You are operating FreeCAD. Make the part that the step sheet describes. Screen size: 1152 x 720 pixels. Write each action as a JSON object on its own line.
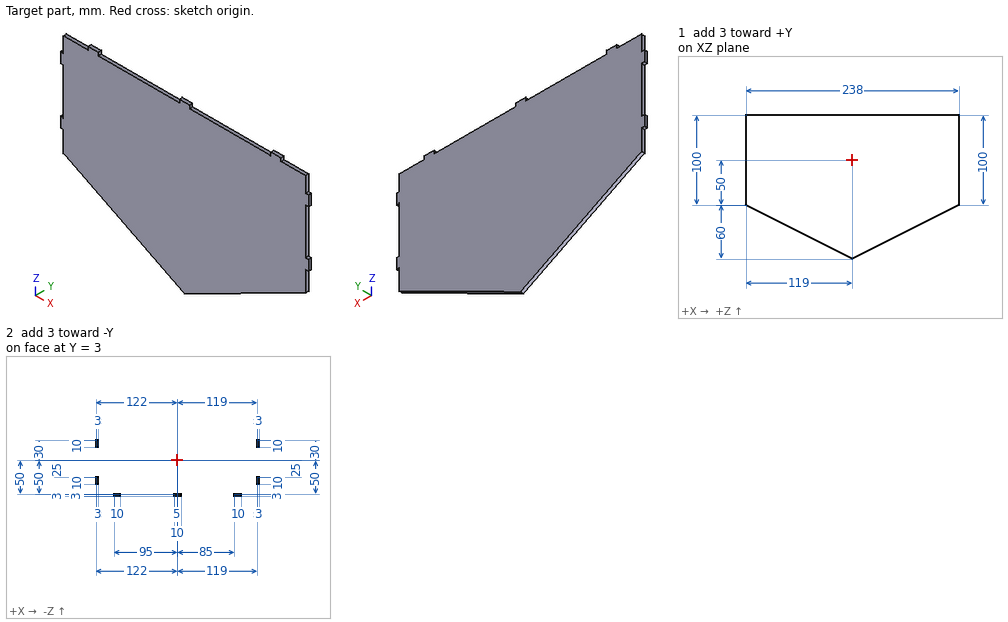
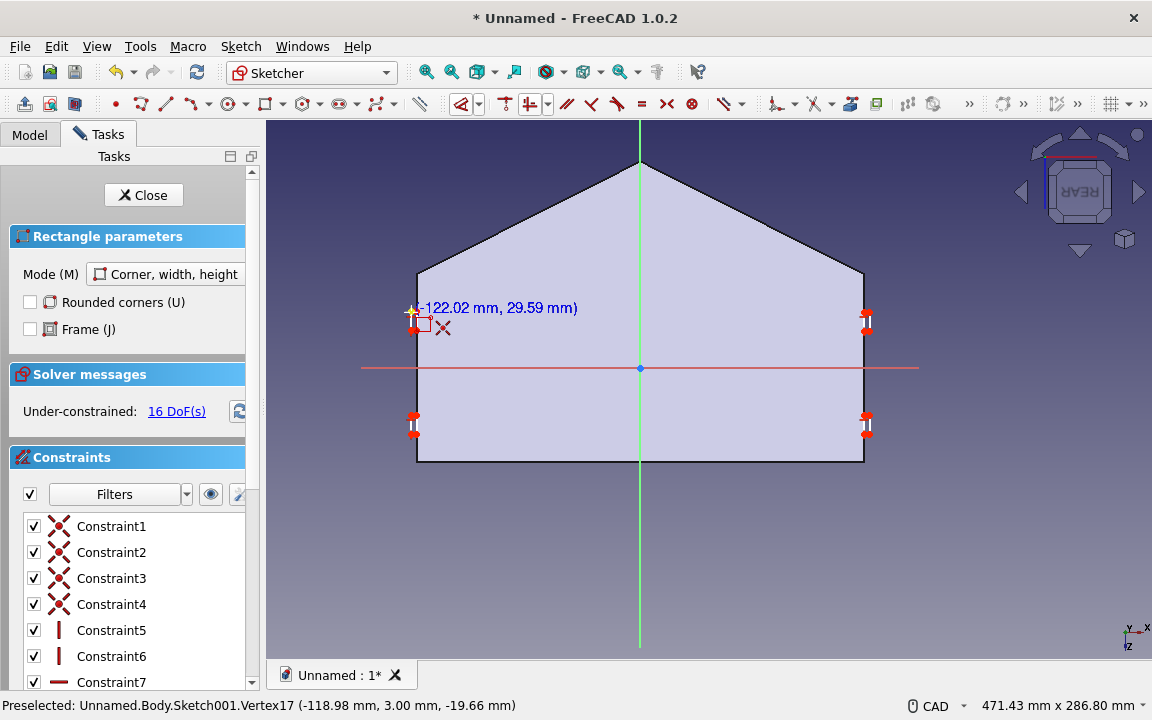
{"action": "scroll", "coordinate": [462, 462], "scroll_direction": "up", "scroll_amount": 6}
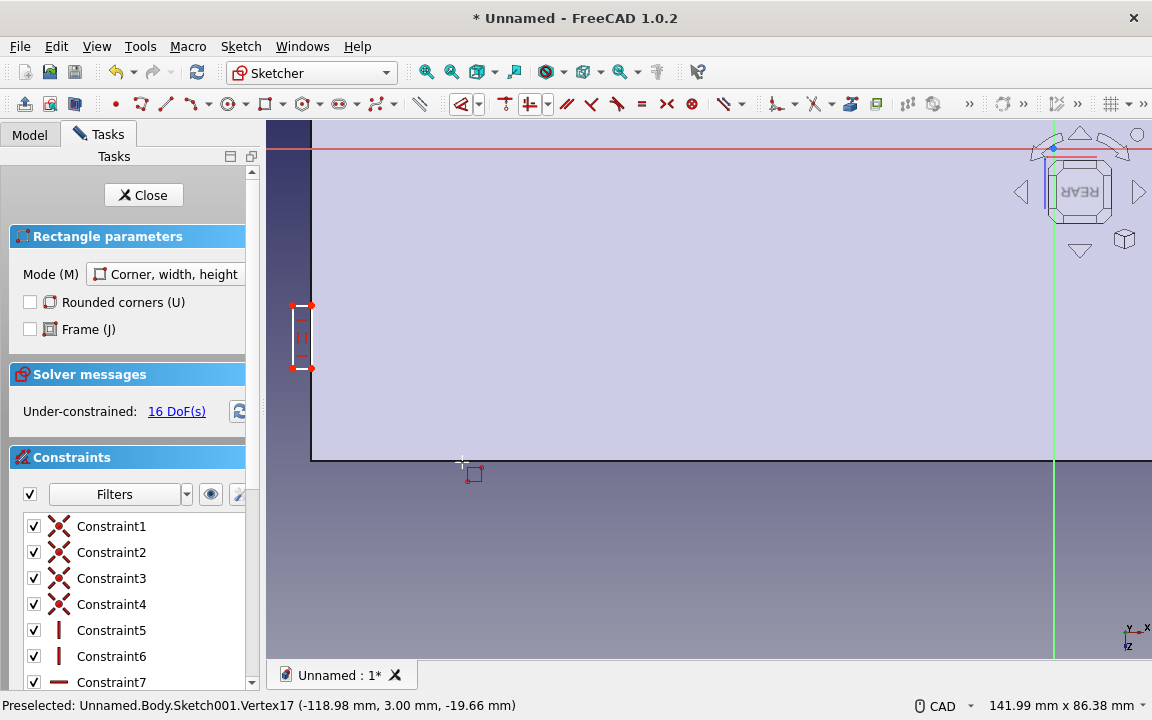
{"action": "left_click", "coordinate": [461, 461]}
{"action": "left_click", "coordinate": [524, 480]}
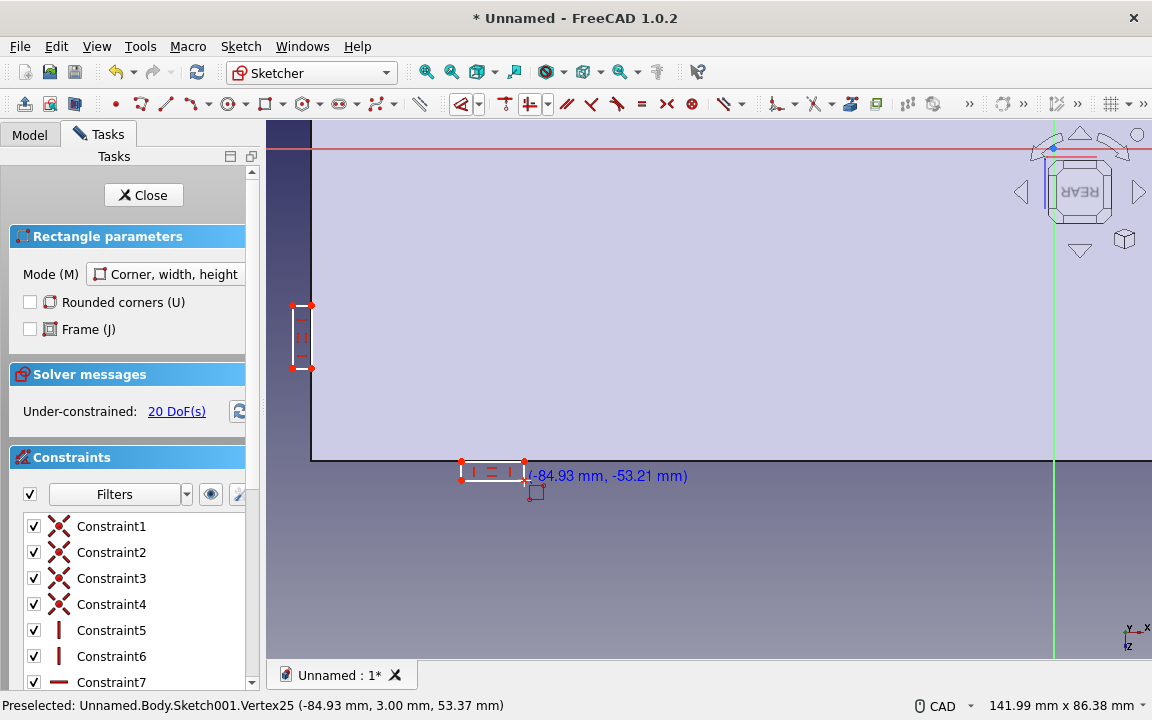
{"action": "scroll", "coordinate": [462, 462], "scroll_direction": "down", "scroll_amount": 6}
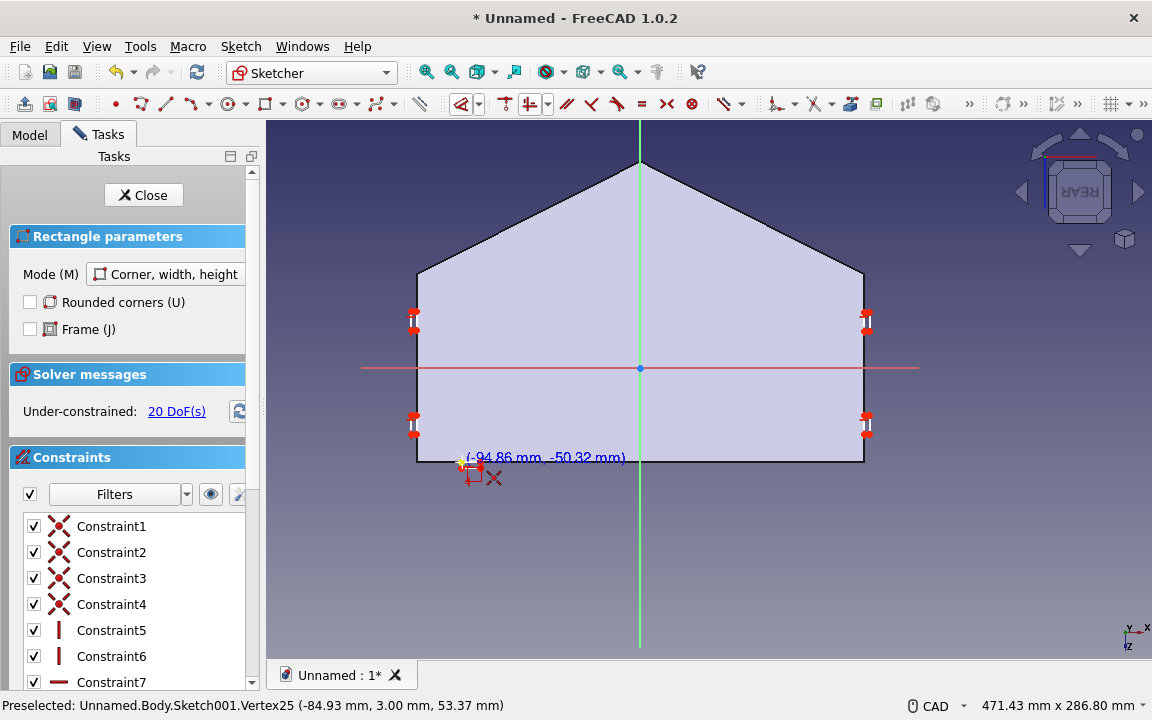
{"action": "scroll", "coordinate": [800, 462], "scroll_direction": "up", "scroll_amount": 6}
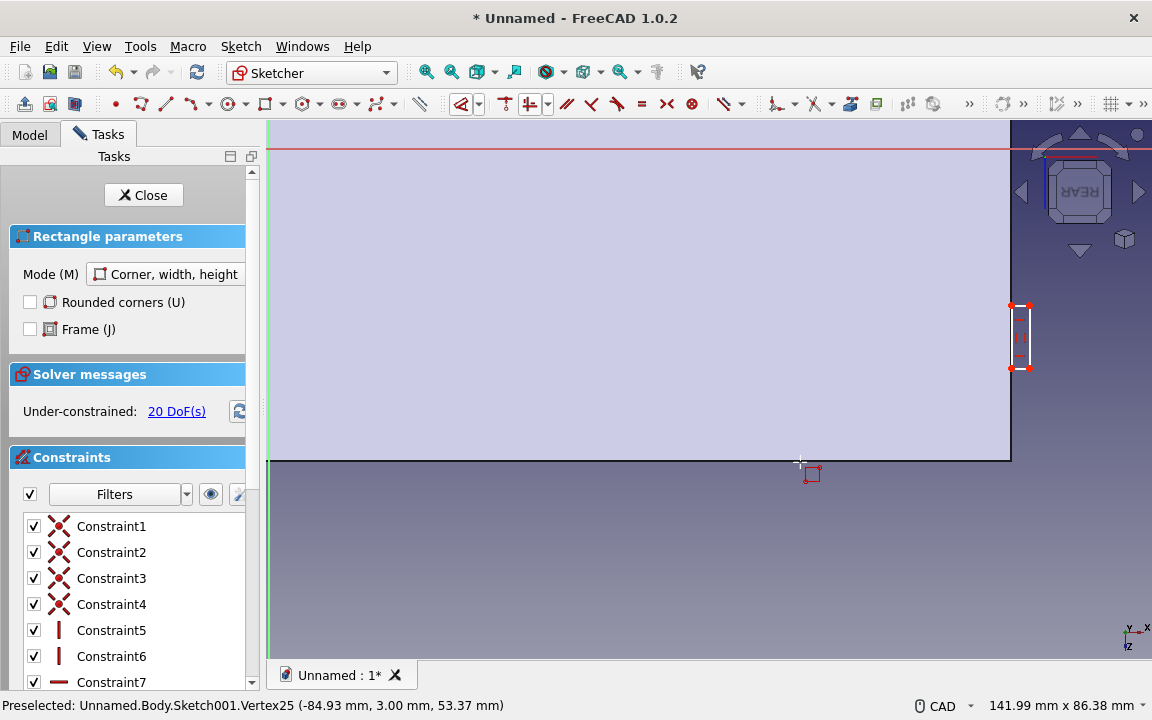
{"action": "left_click", "coordinate": [799, 461]}
{"action": "left_click", "coordinate": [862, 480]}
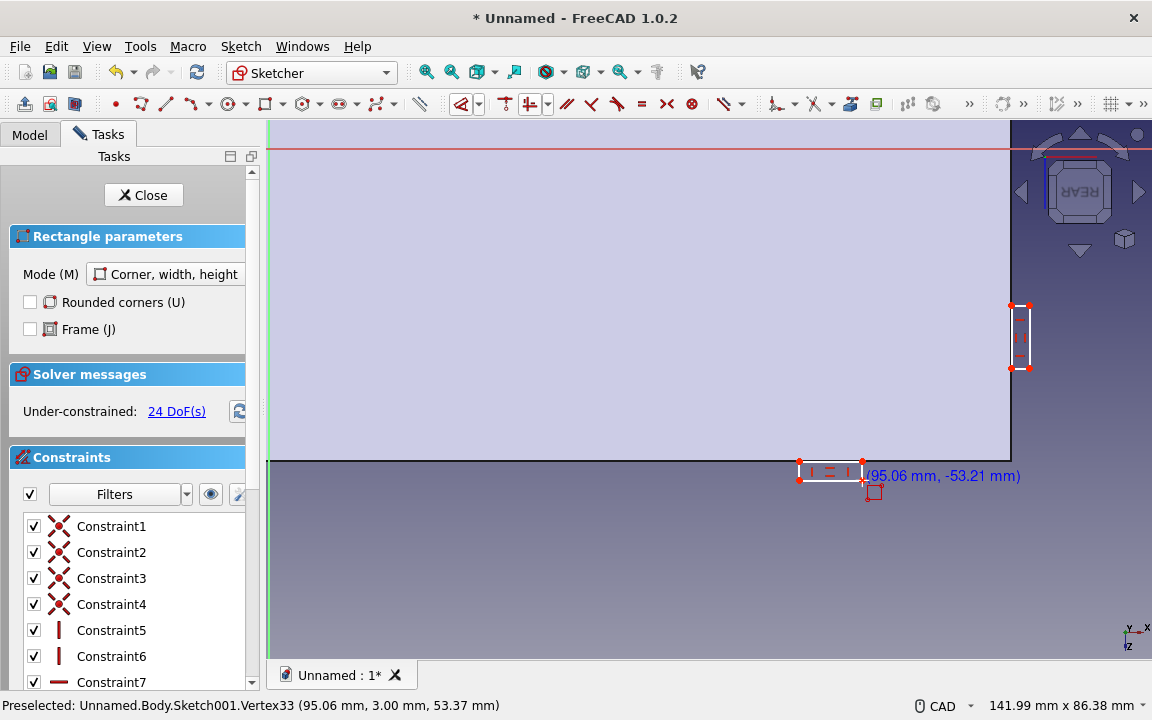
{"action": "scroll", "coordinate": [801, 462], "scroll_direction": "down", "scroll_amount": 6}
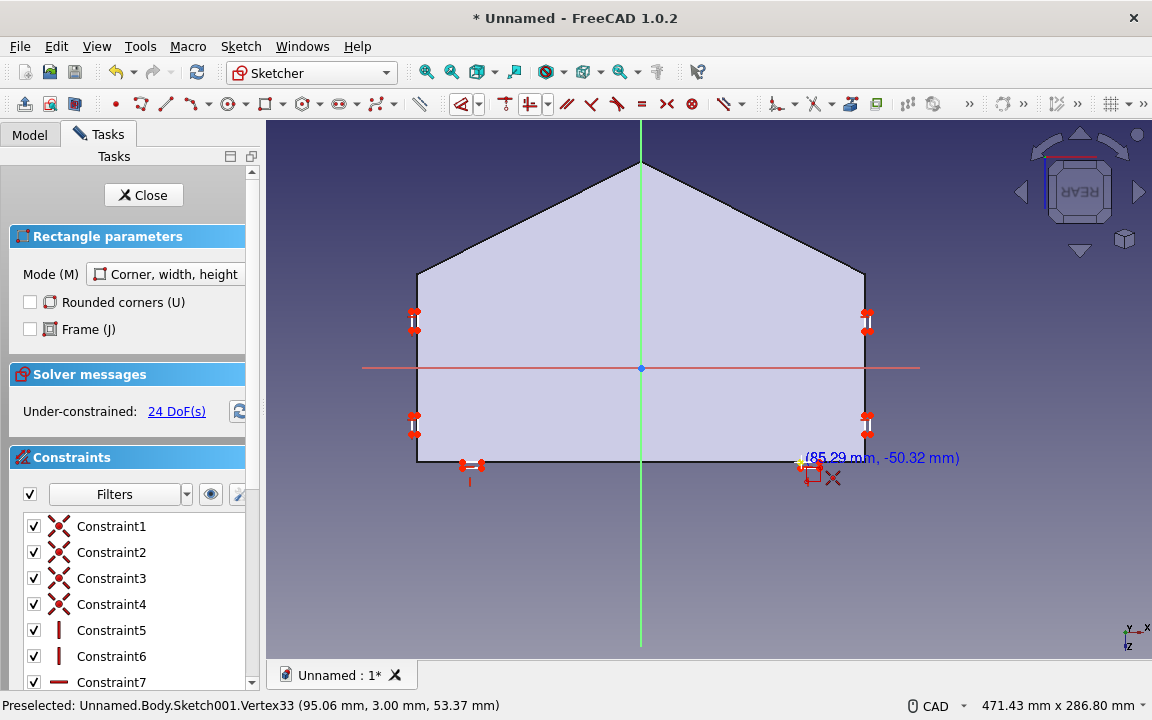
{"action": "scroll", "coordinate": [632, 462], "scroll_direction": "up", "scroll_amount": 6}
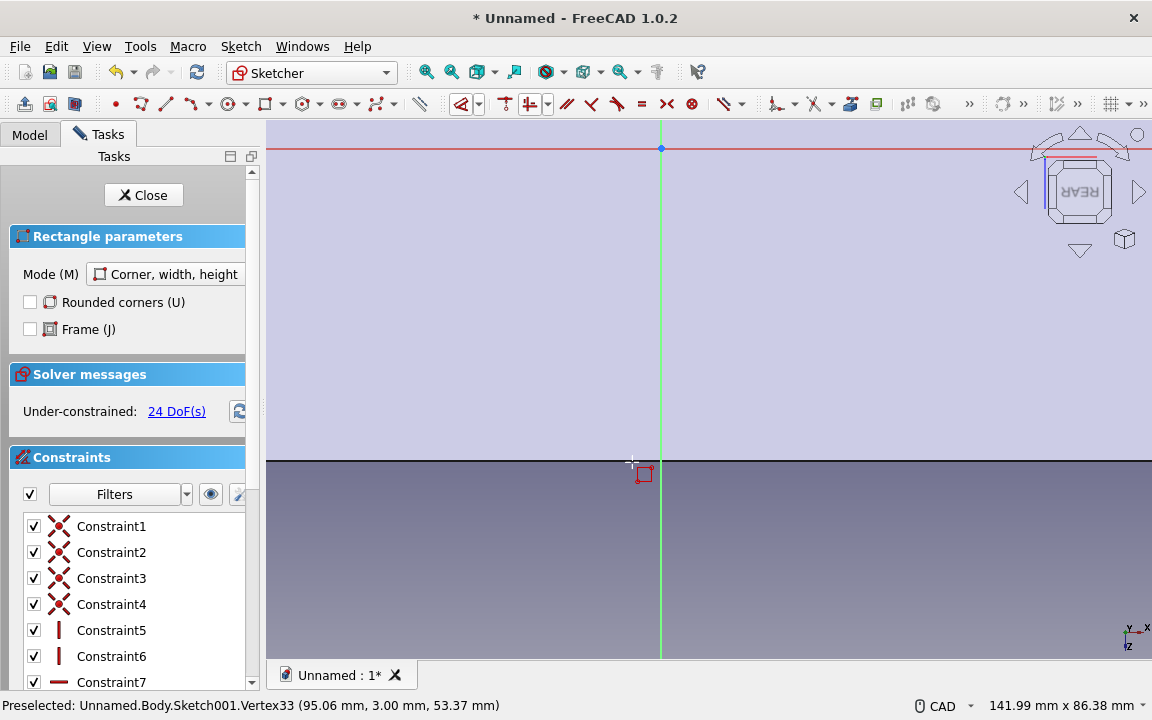
{"action": "left_click", "coordinate": [630, 461]}
{"action": "left_click", "coordinate": [693, 480]}
{"action": "key", "text": "Escape"}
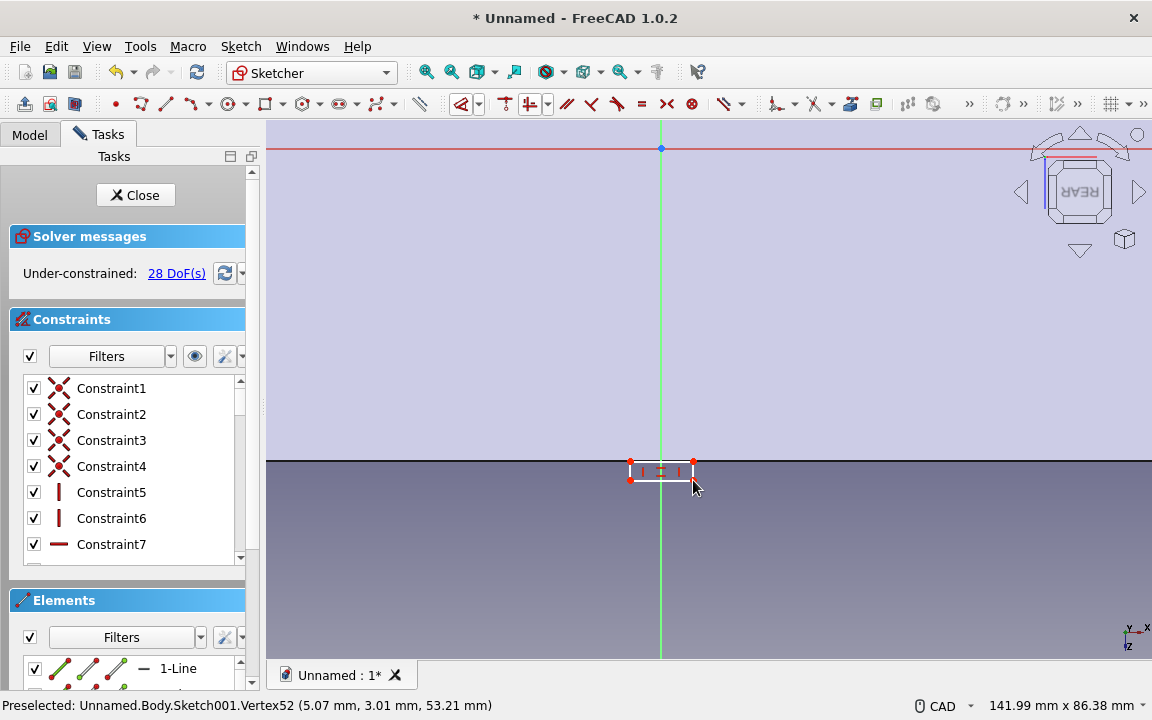
{"action": "scroll", "coordinate": [631, 462], "scroll_direction": "down", "scroll_amount": 6}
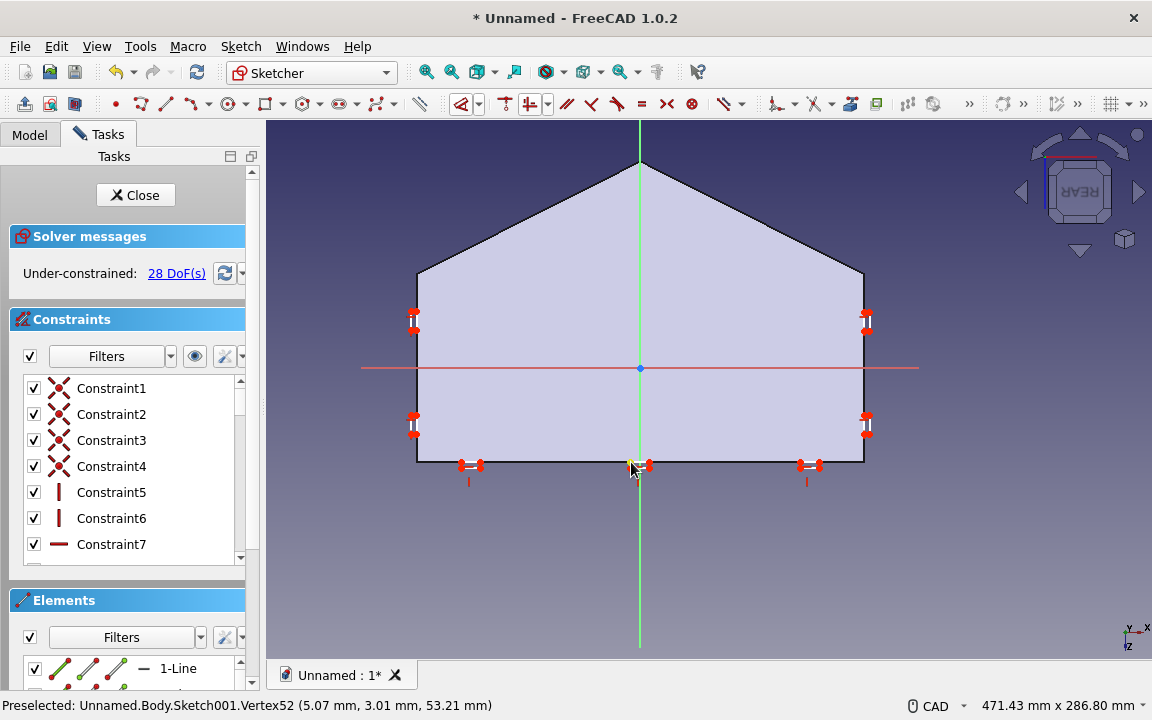
{"action": "scroll", "coordinate": [867, 331], "scroll_direction": "up", "scroll_amount": 10}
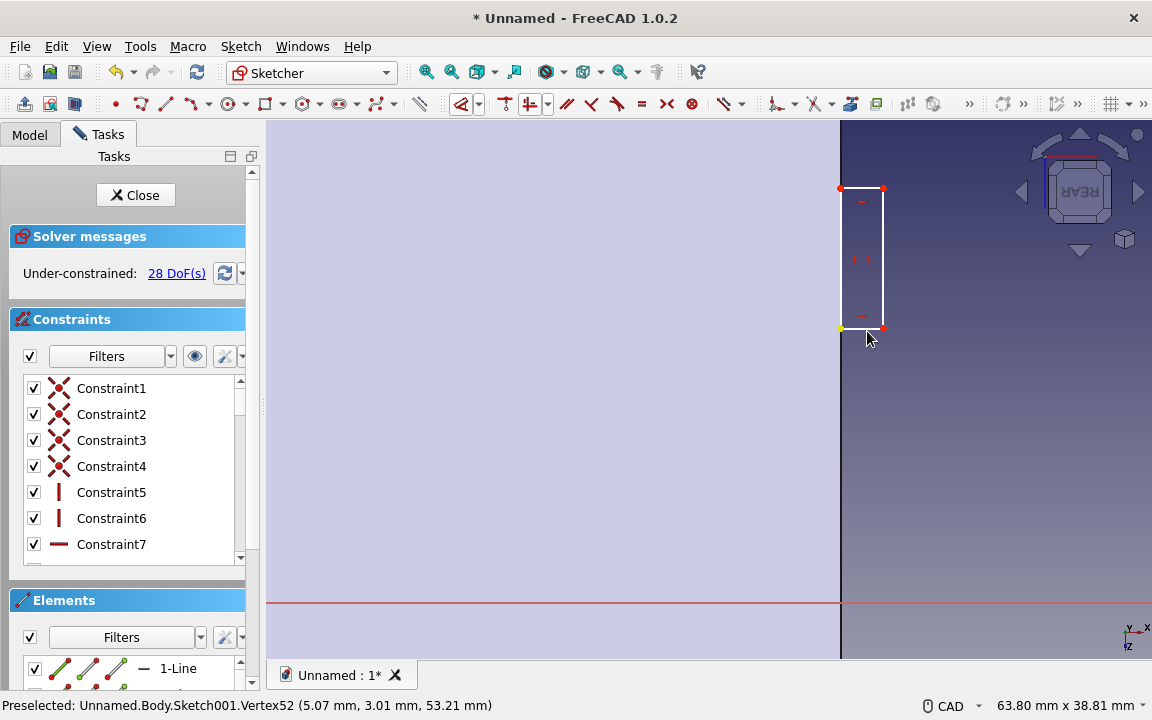
{"action": "left_click", "coordinate": [862, 329]}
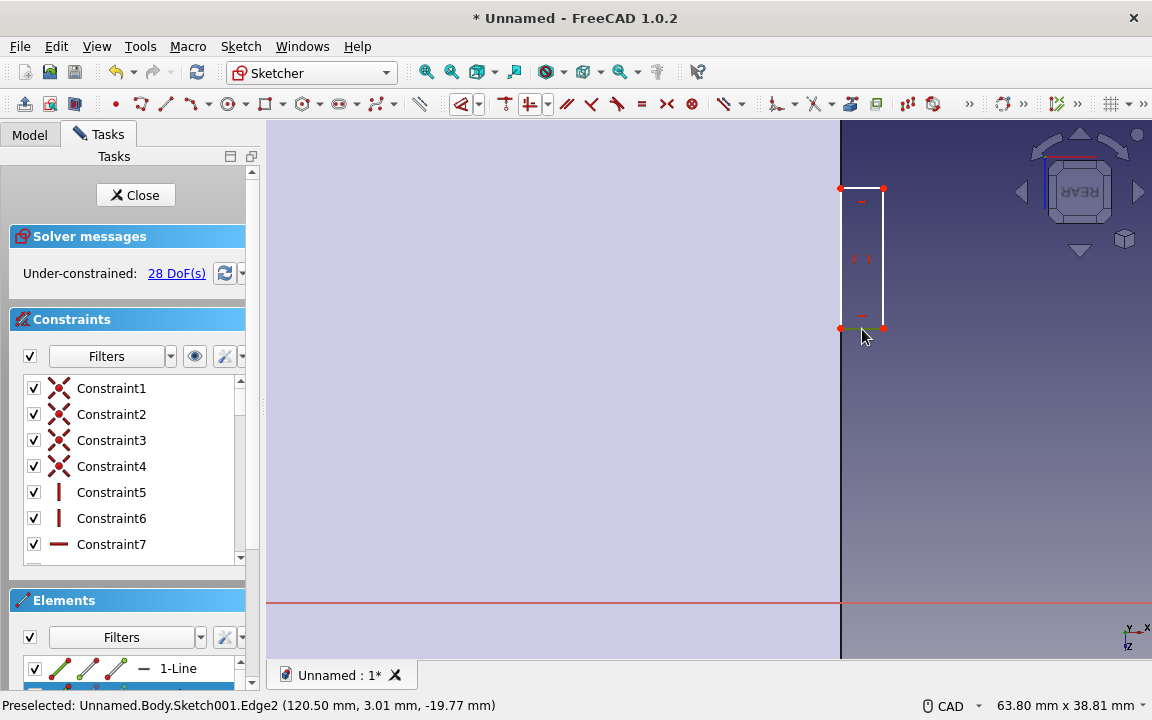
{"action": "key", "text": "l"}